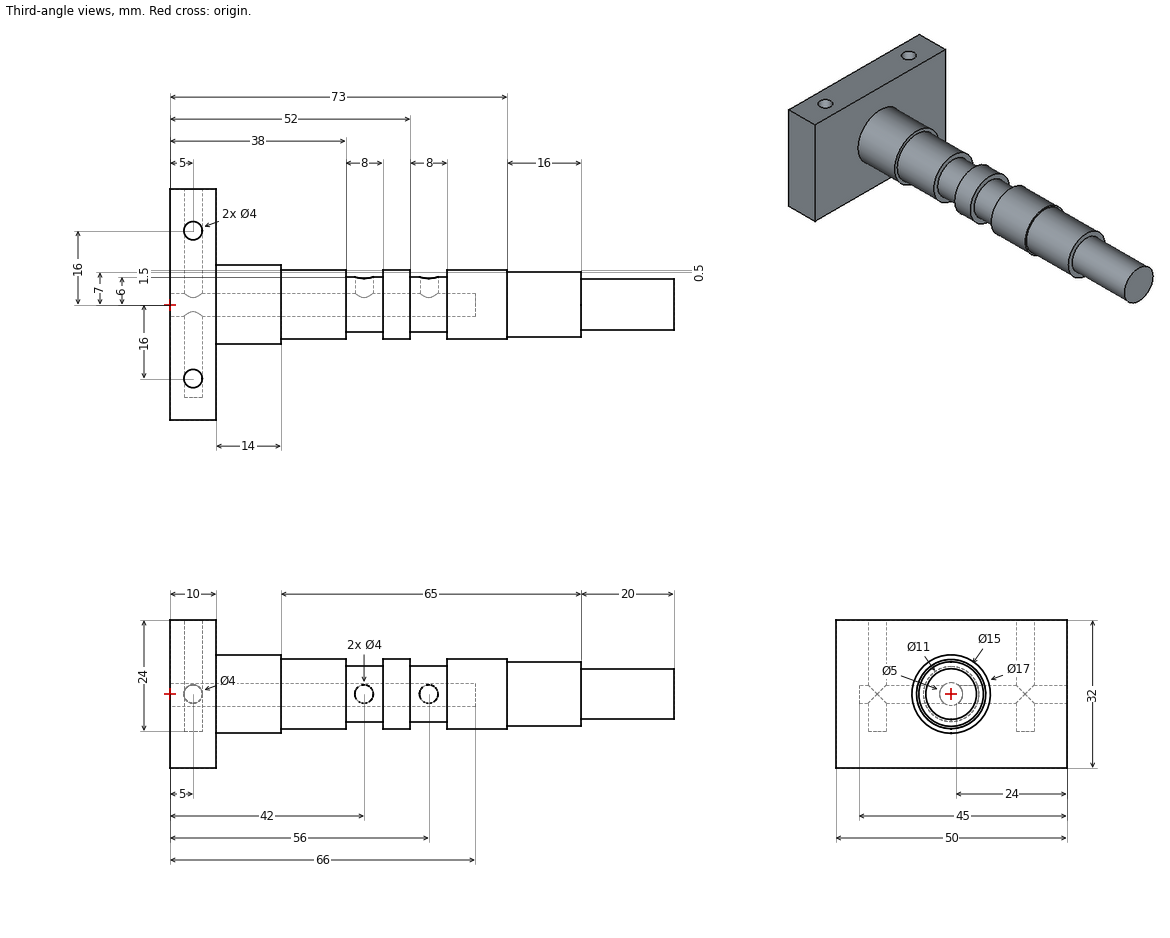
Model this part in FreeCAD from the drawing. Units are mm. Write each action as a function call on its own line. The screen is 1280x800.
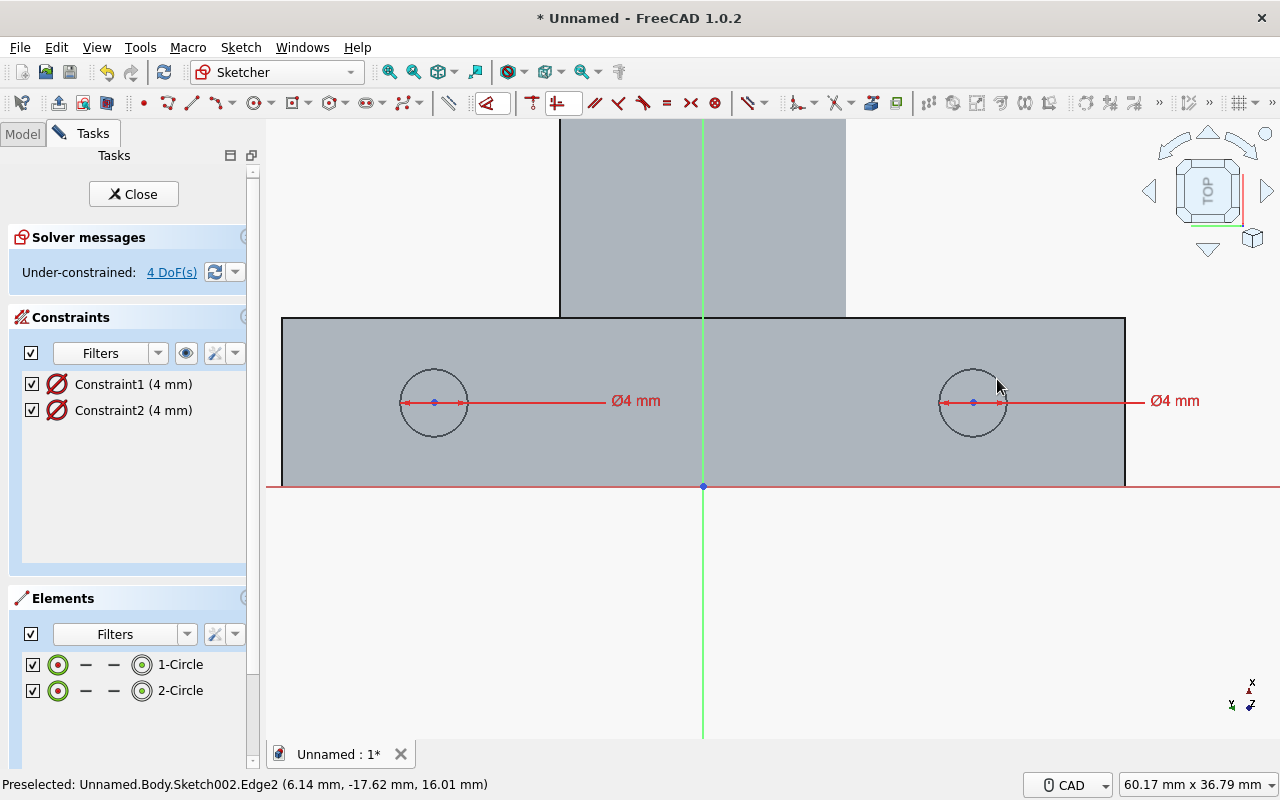
click(434, 403)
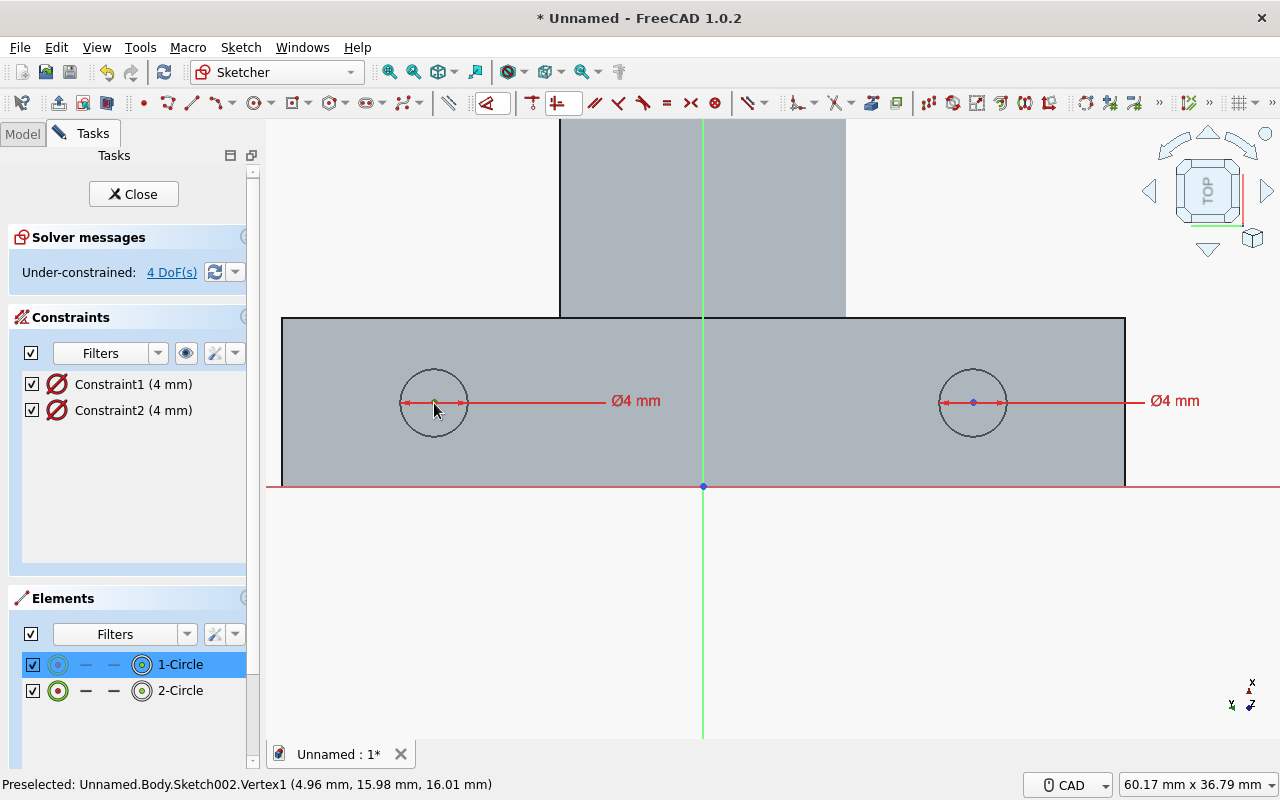
click(973, 403)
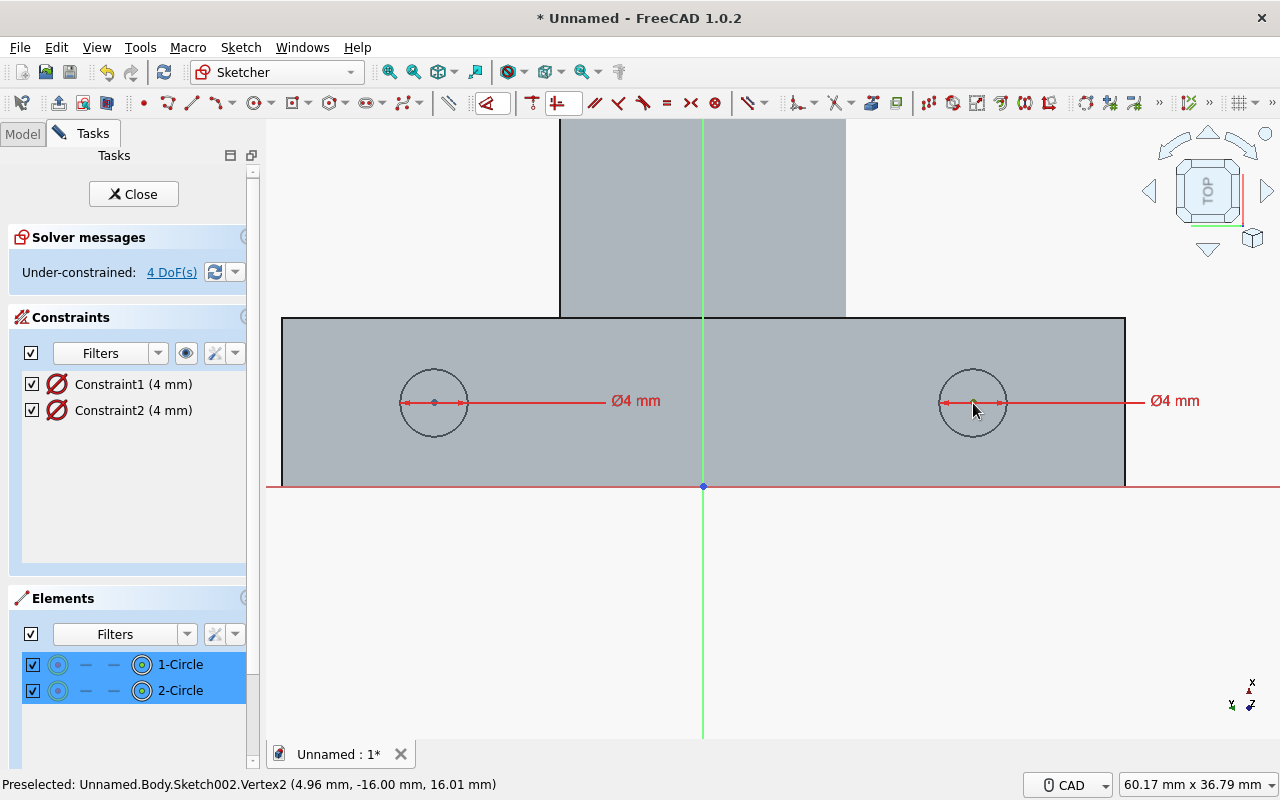
click(576, 104)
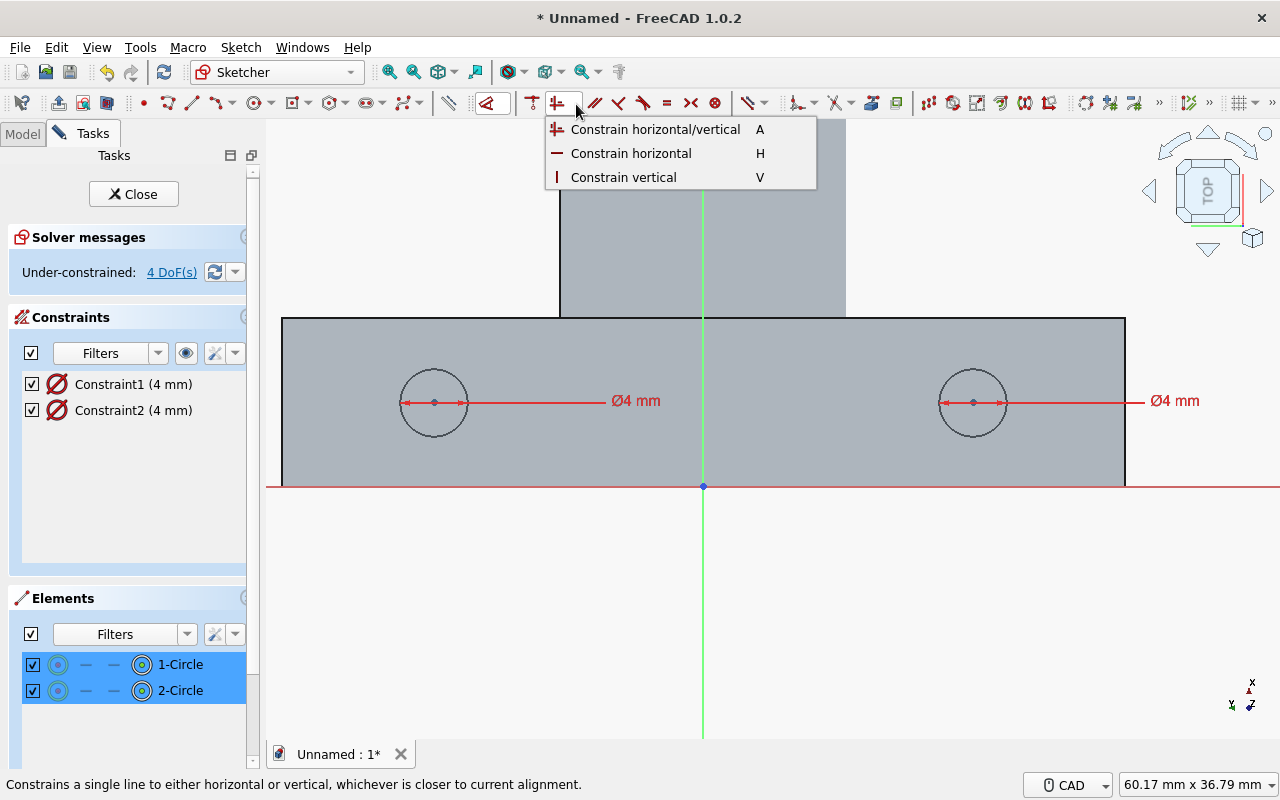
click(681, 153)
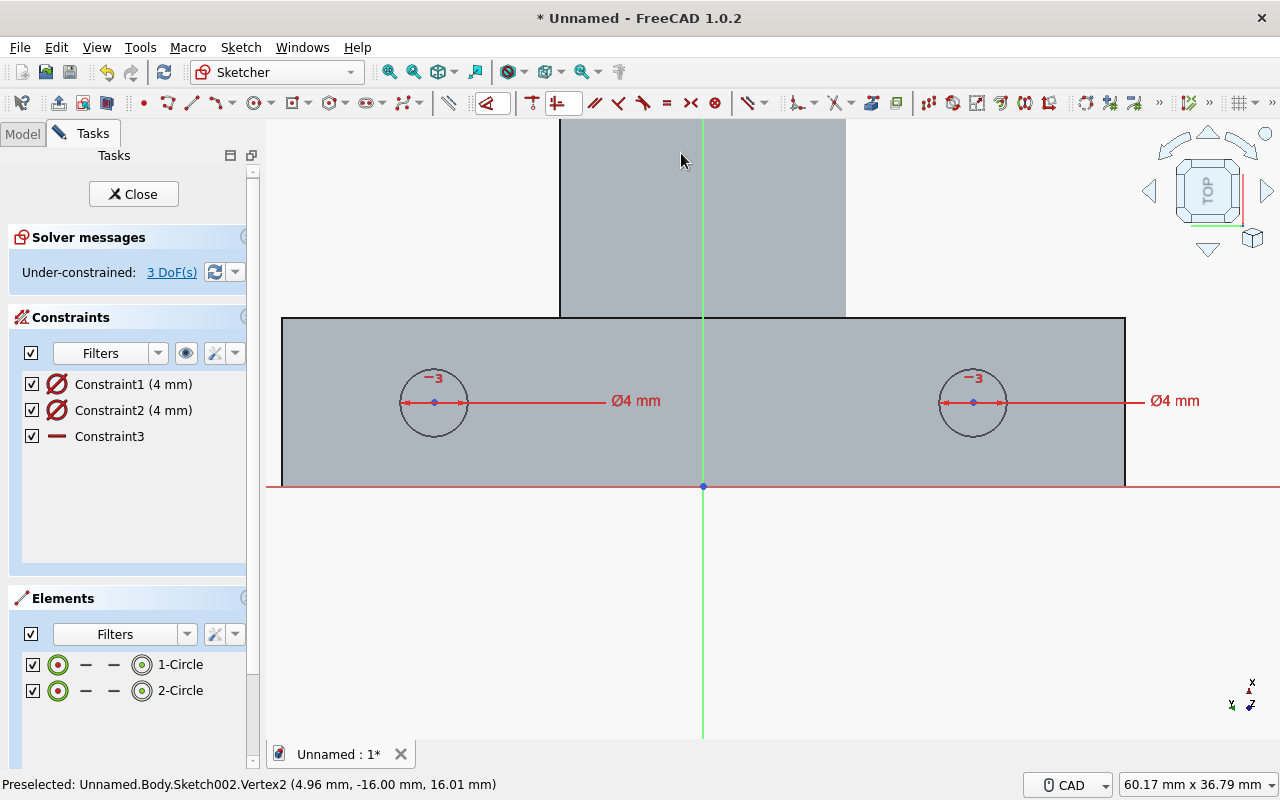
click(486, 104)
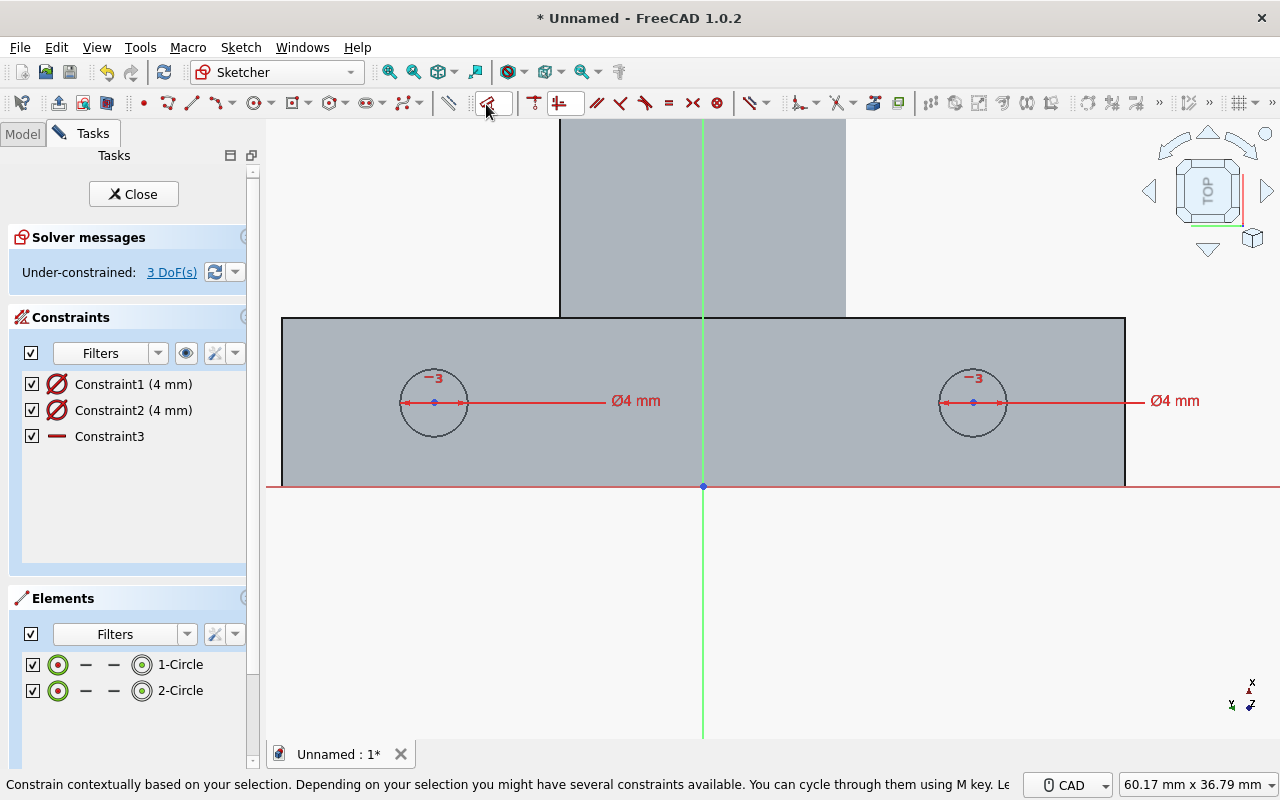
click(434, 403)
click(400, 445)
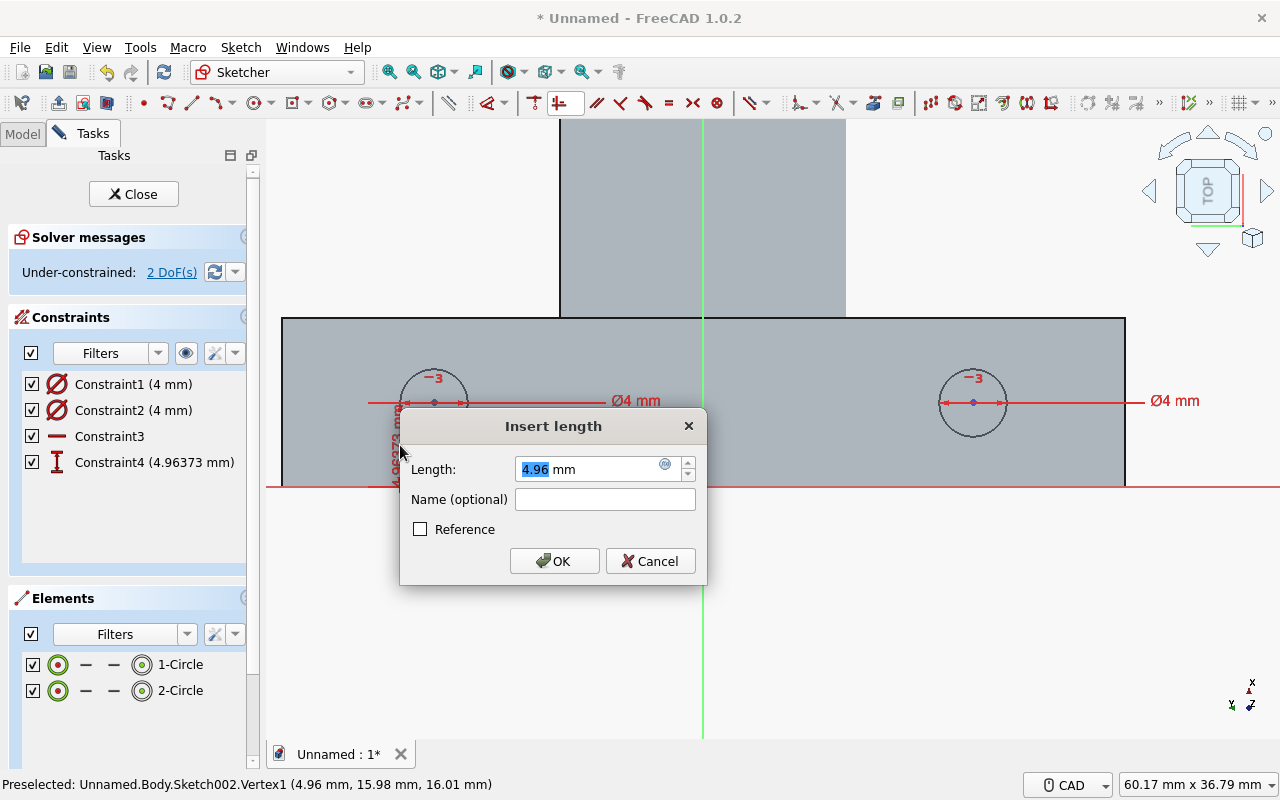
text(5)
key(Return)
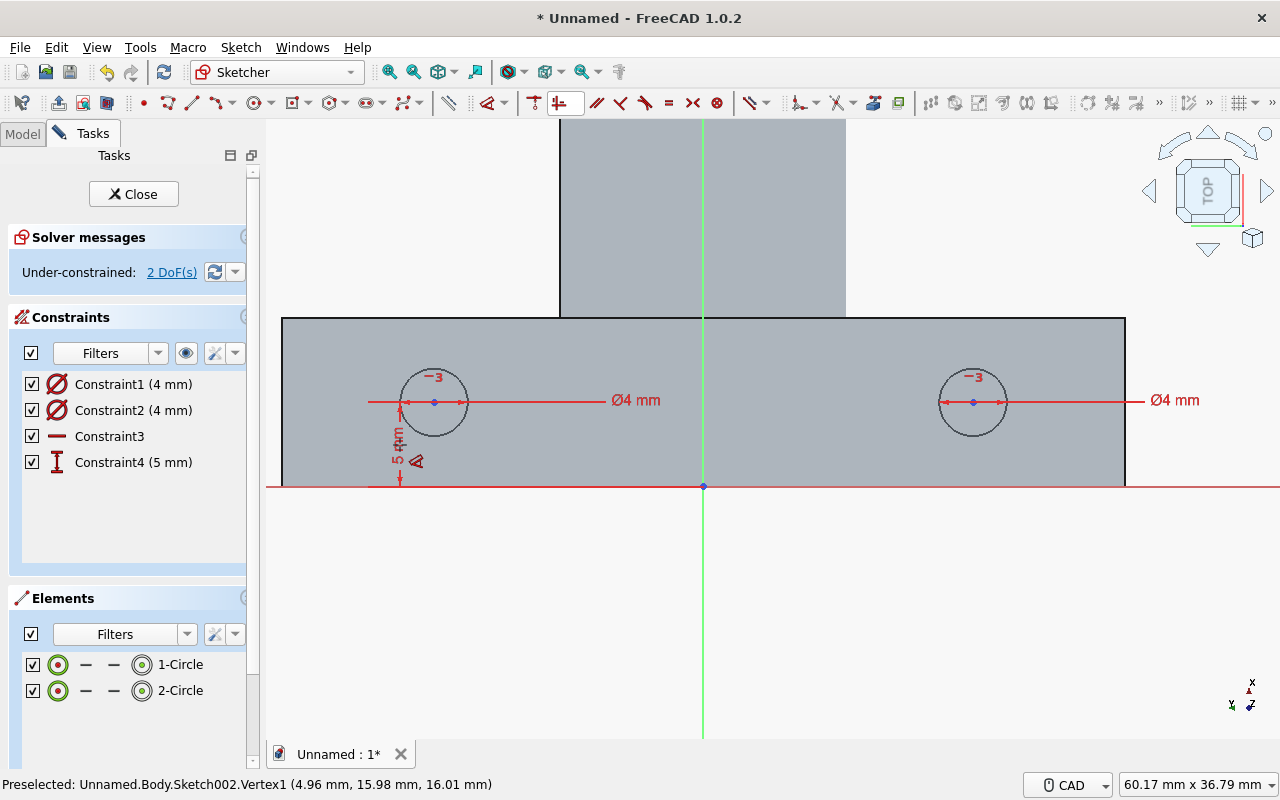
click(434, 402)
click(569, 521)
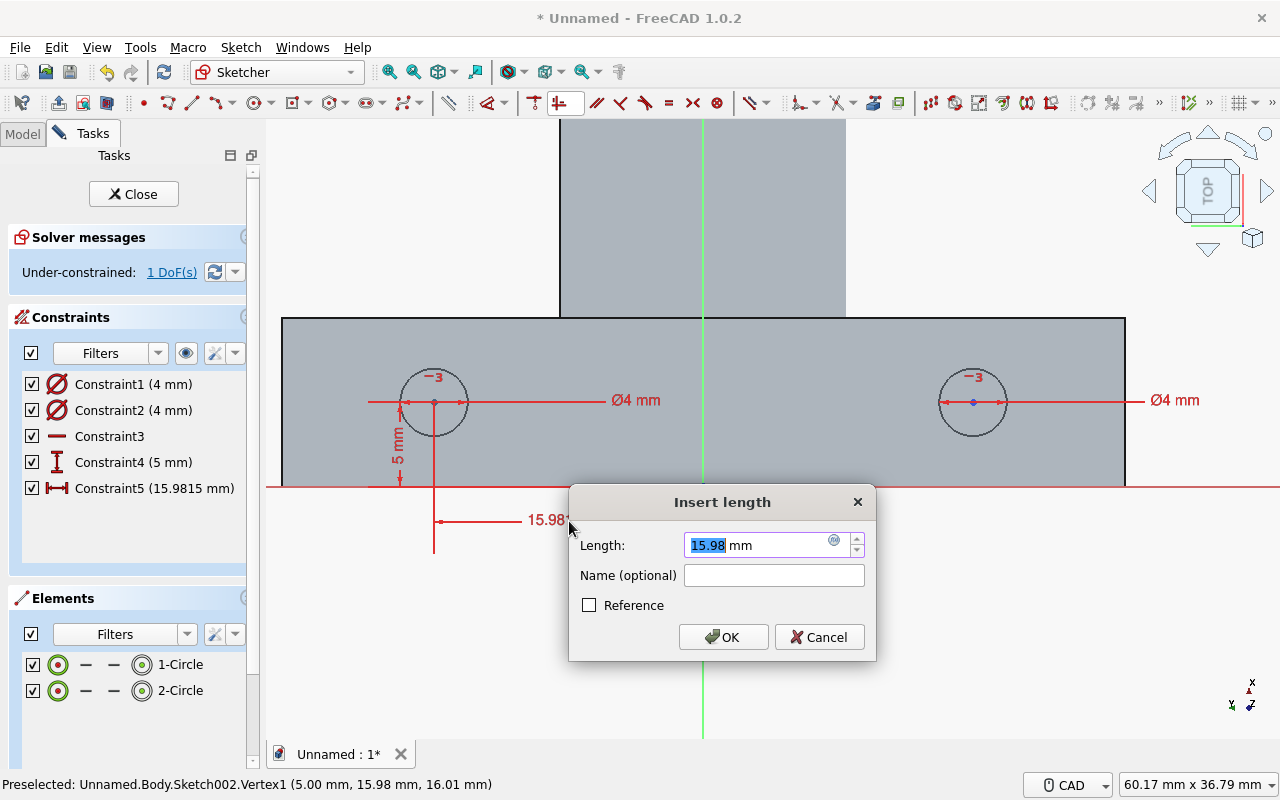
text(16)
key(Return)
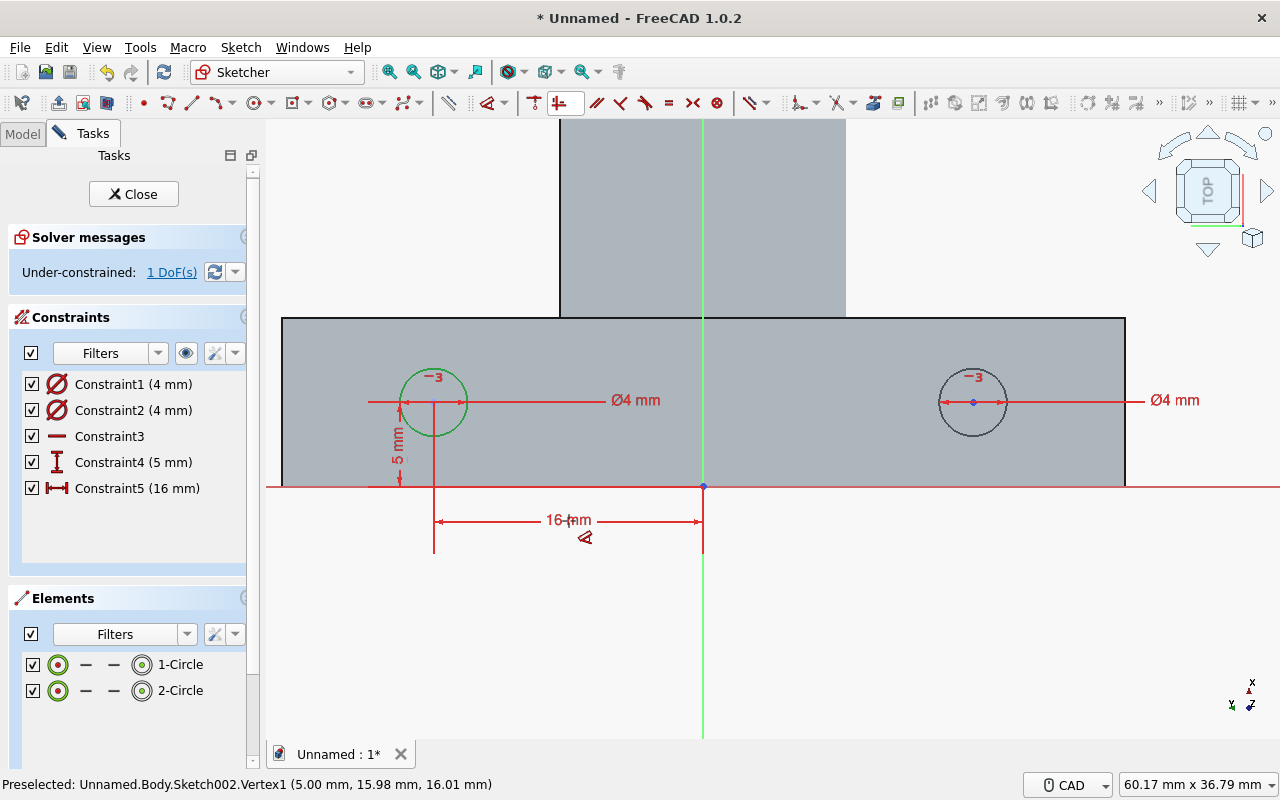
click(973, 402)
click(838, 521)